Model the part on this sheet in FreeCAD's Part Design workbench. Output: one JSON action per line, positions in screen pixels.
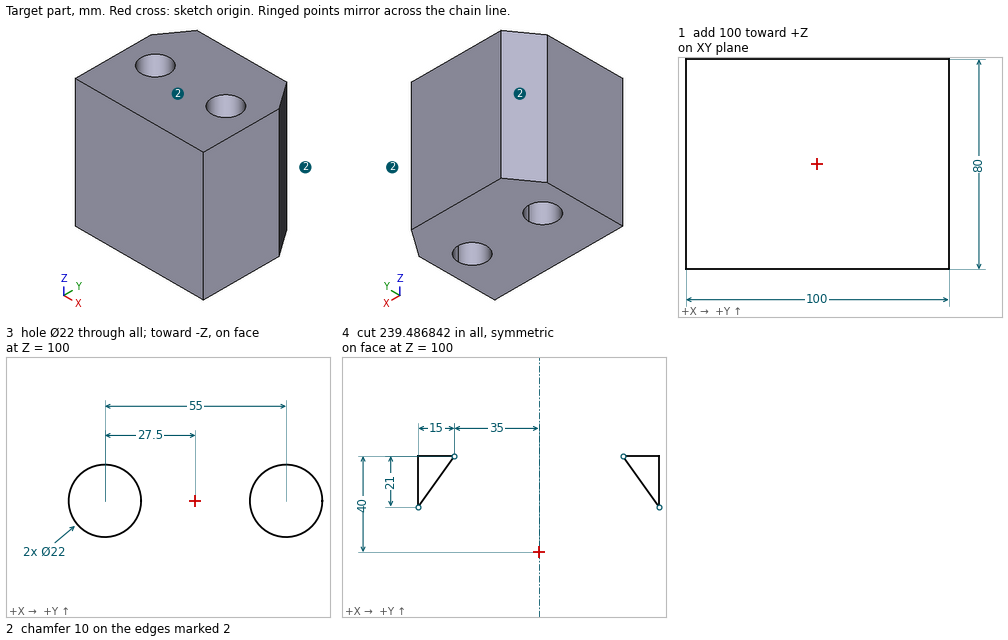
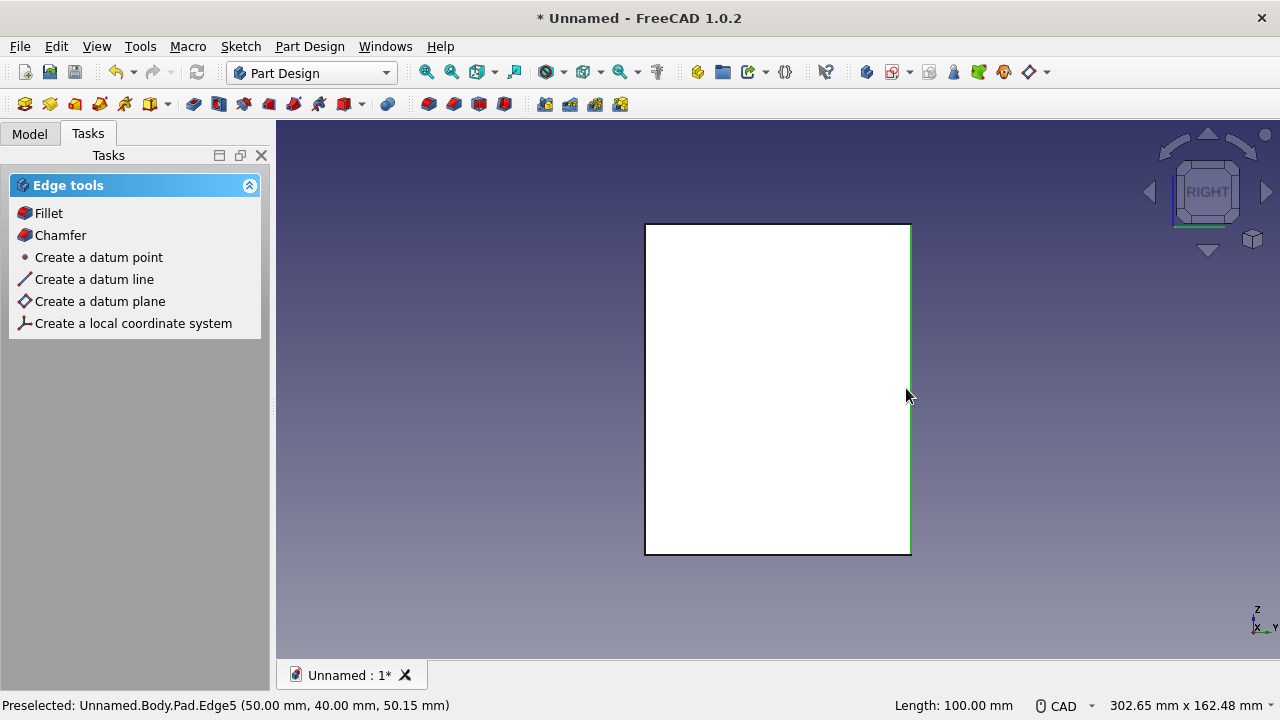
{"action": "key", "text": "5"}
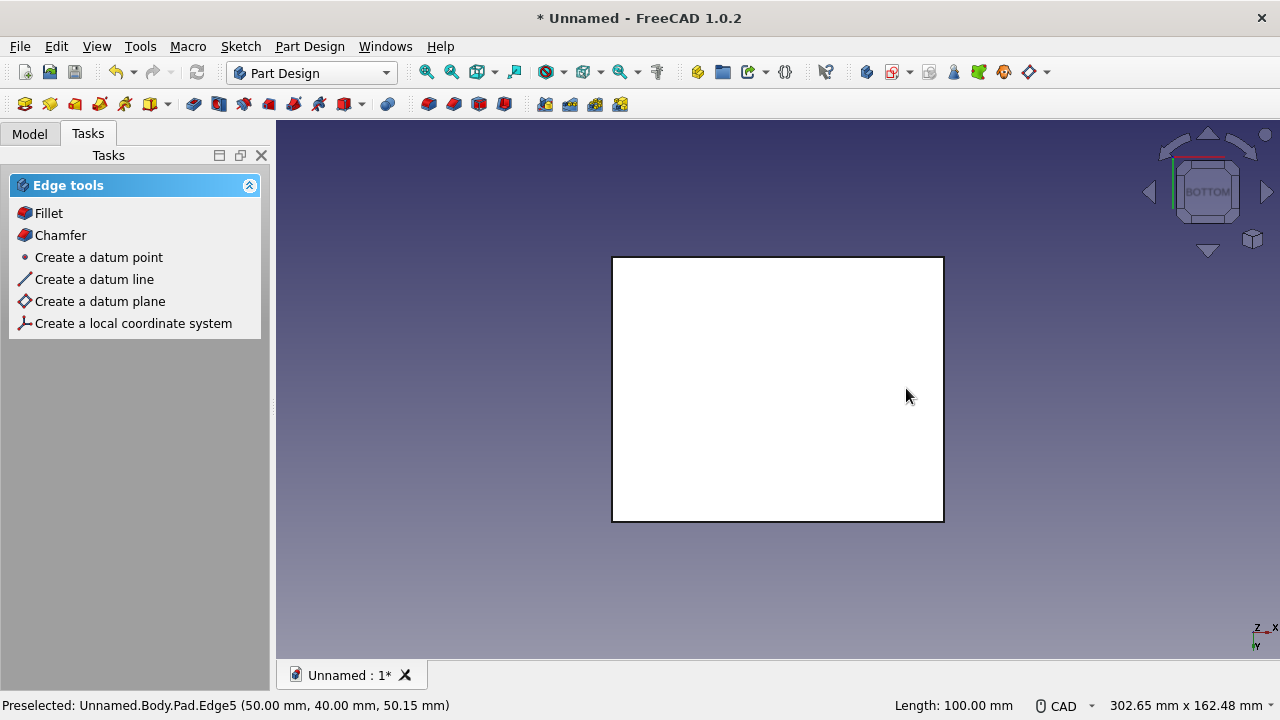
{"action": "key", "text": "4"}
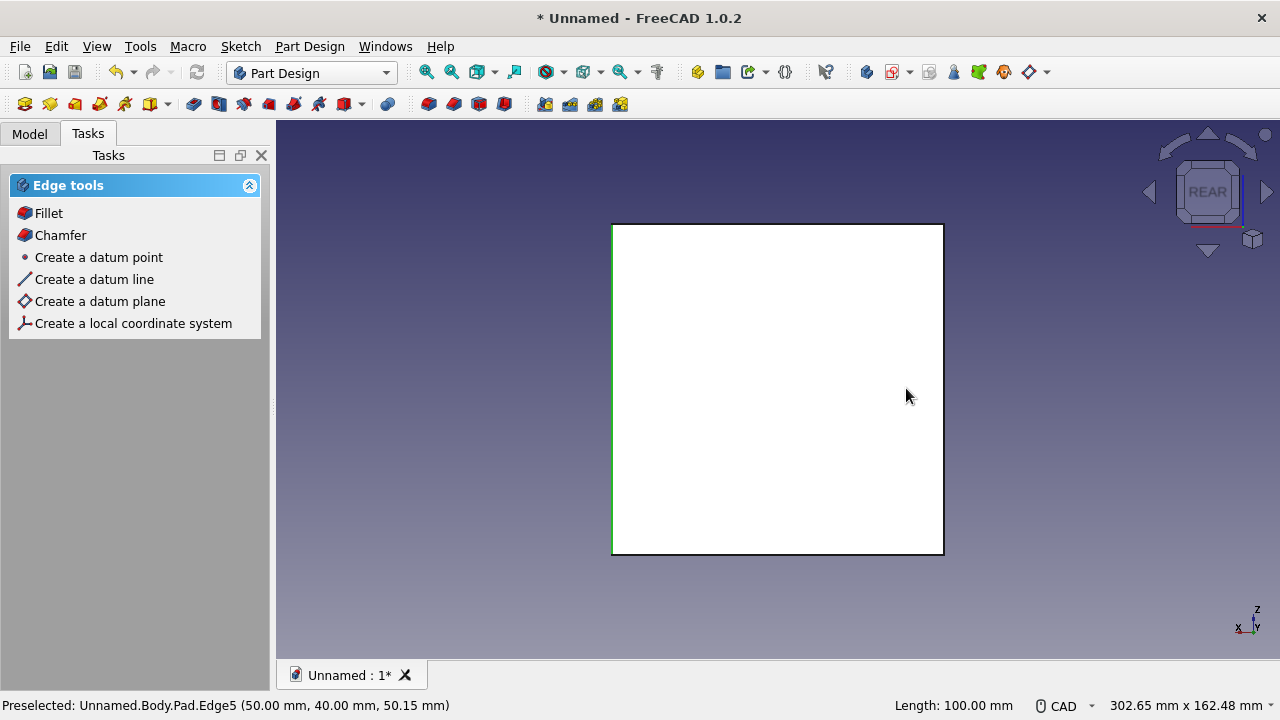
{"action": "left_click", "coordinate": [944, 388], "text": "ctrl"}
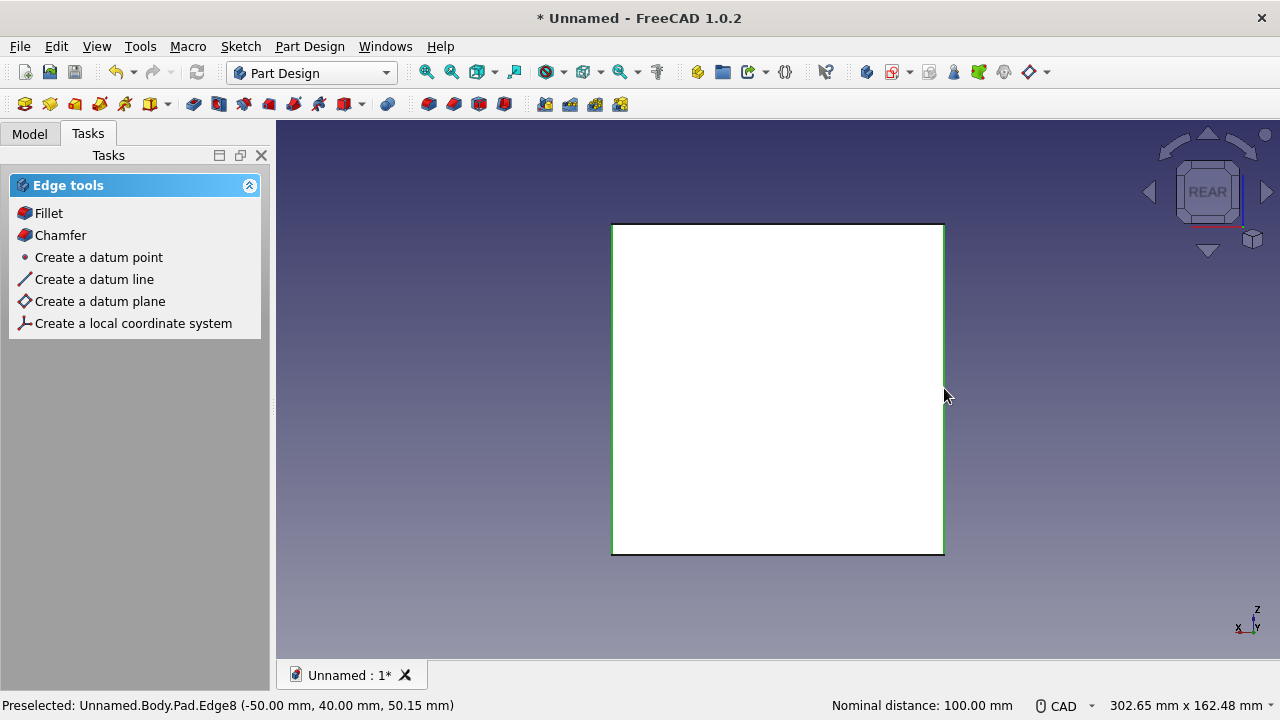
{"action": "left_click", "coordinate": [454, 104]}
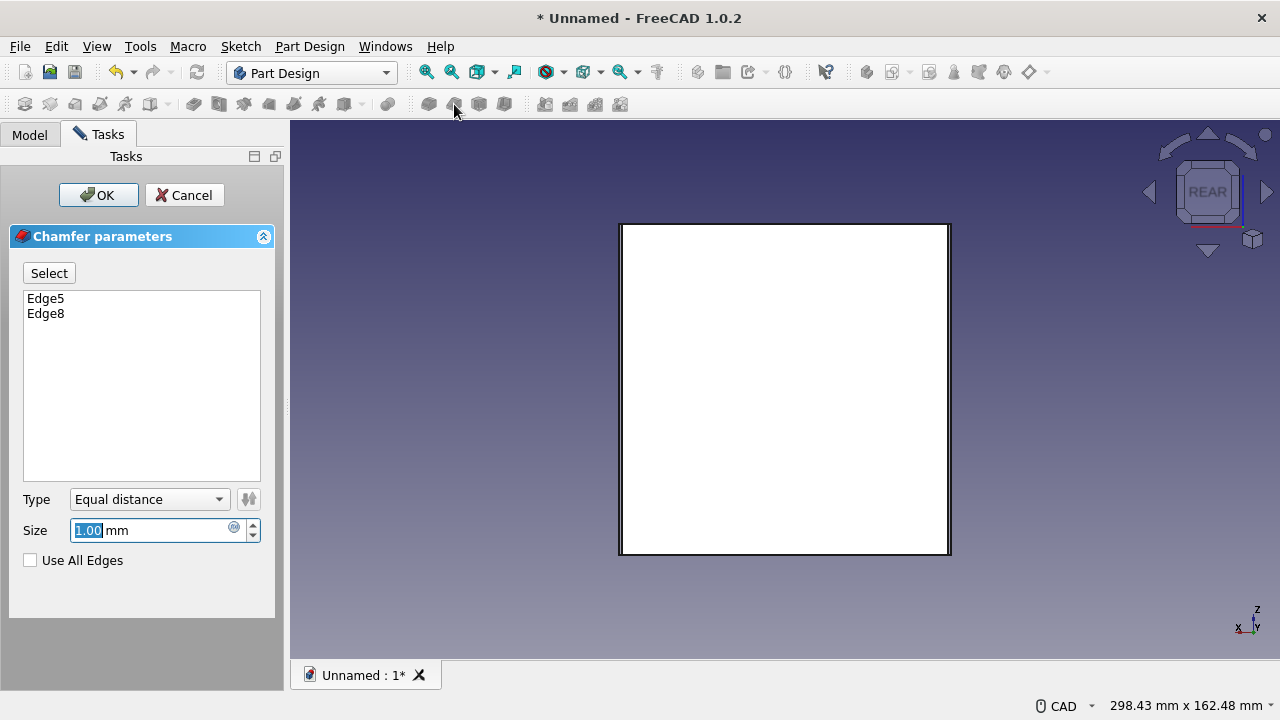
{"action": "type", "text": "10"}
{"action": "key", "text": "Tab"}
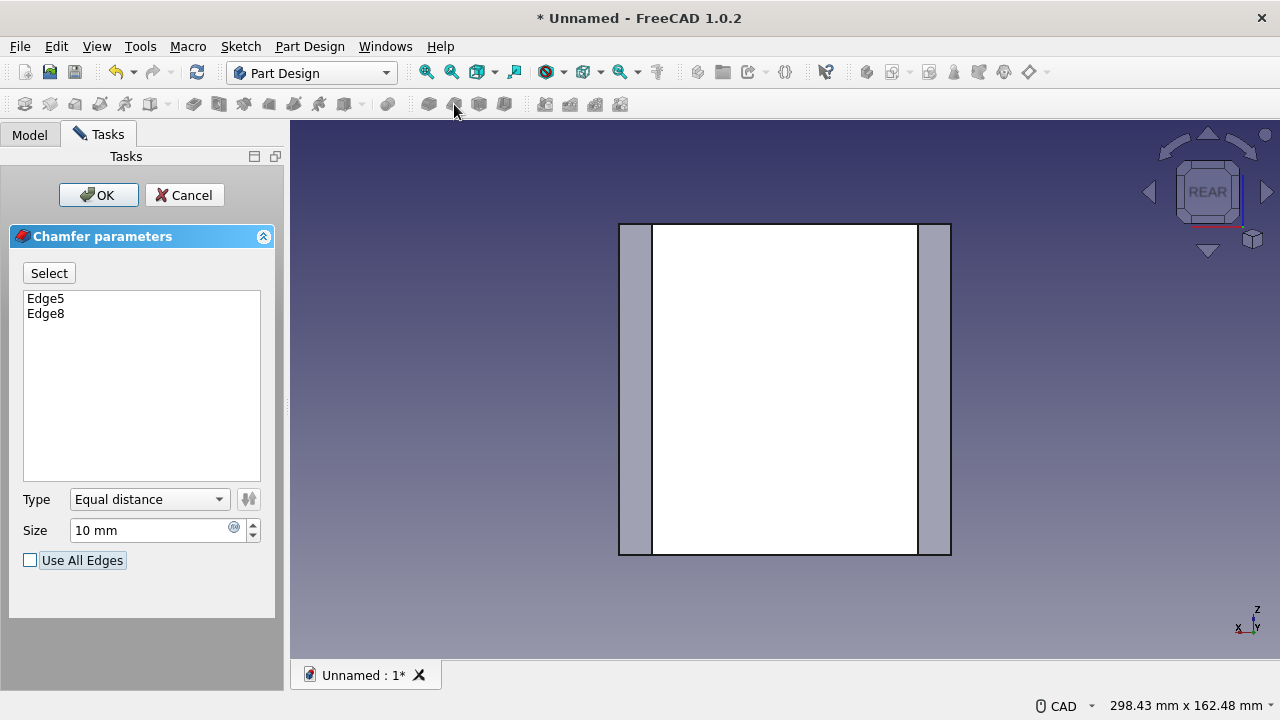
{"action": "left_click", "coordinate": [99, 195]}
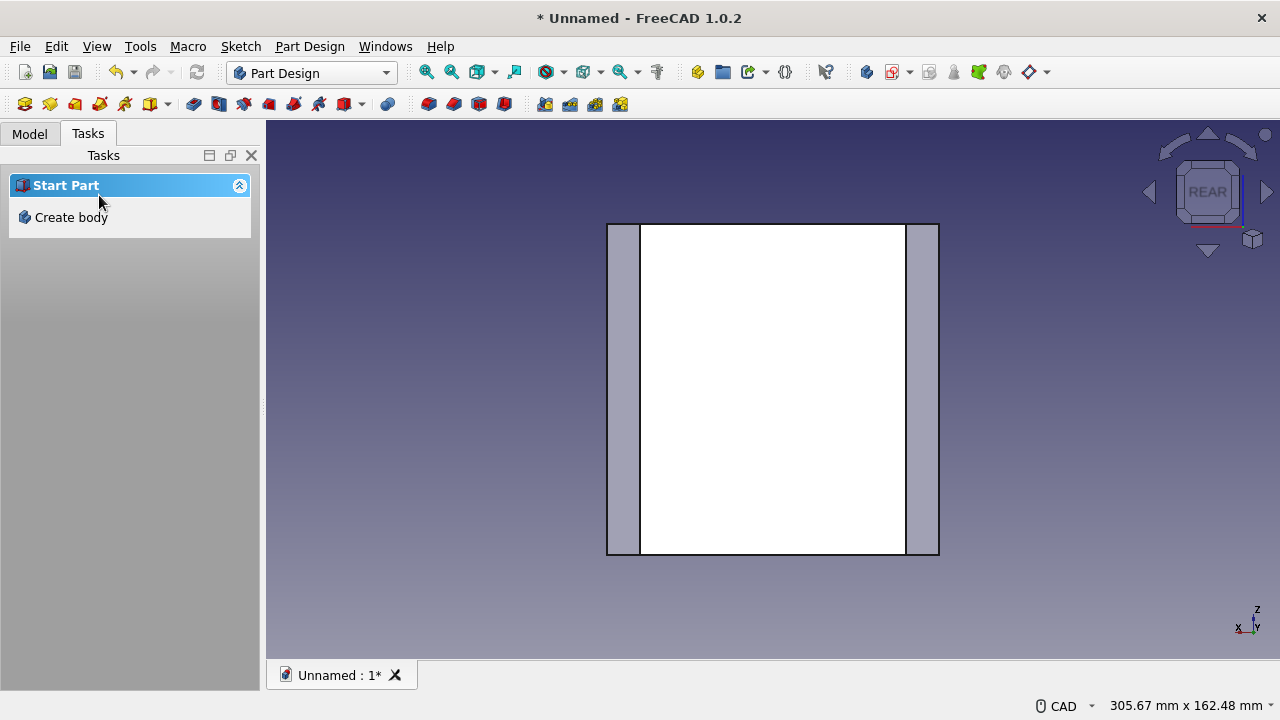
{"action": "key", "text": "0"}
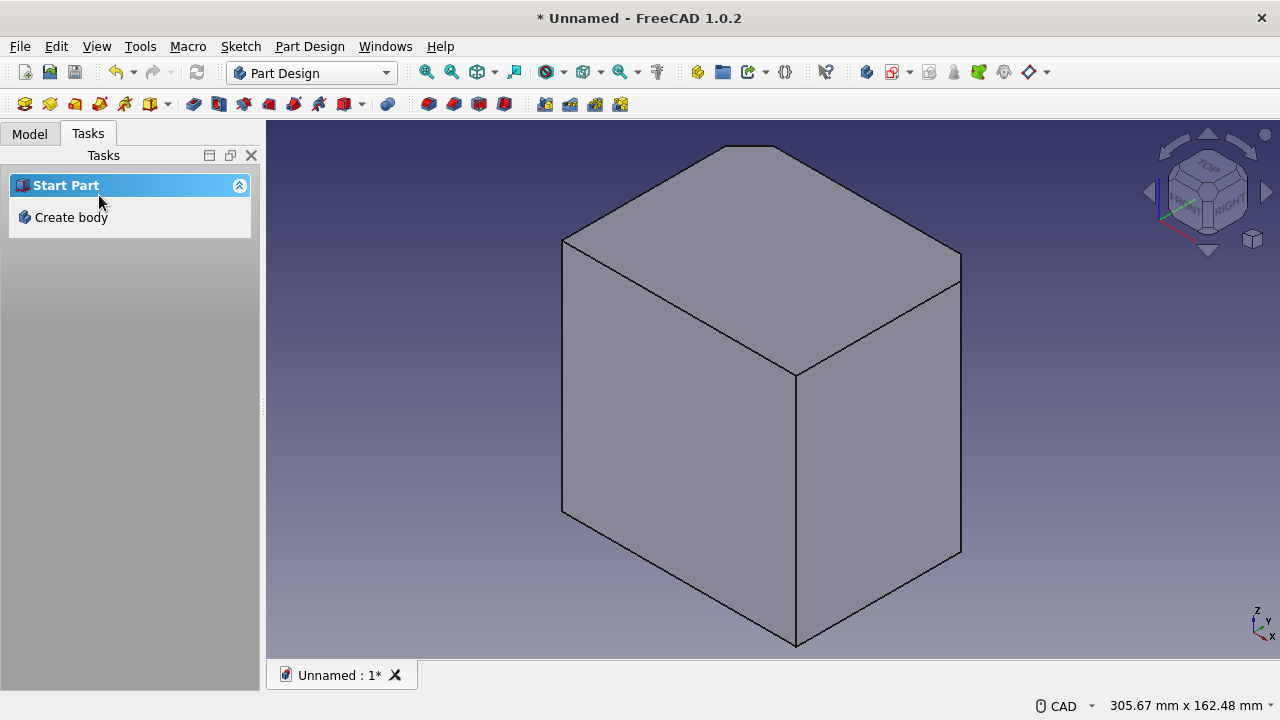
{"action": "left_click", "coordinate": [773, 253]}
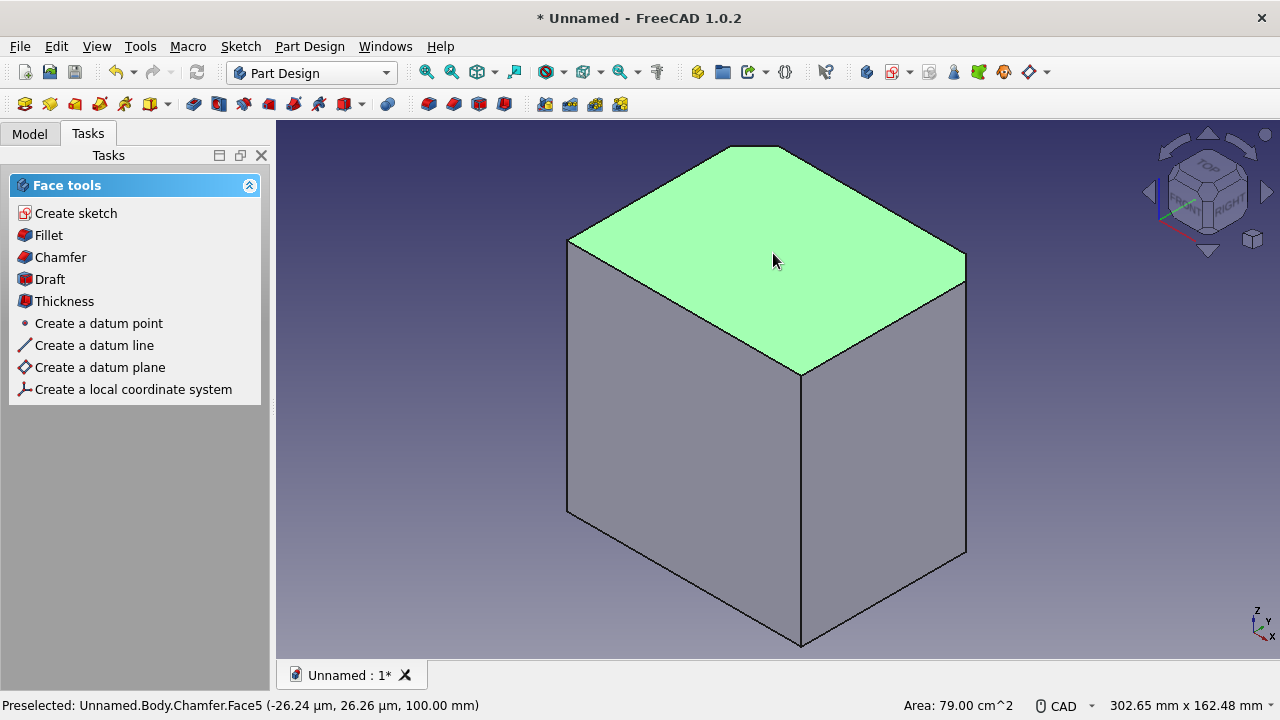
{"action": "left_click", "coordinate": [892, 72]}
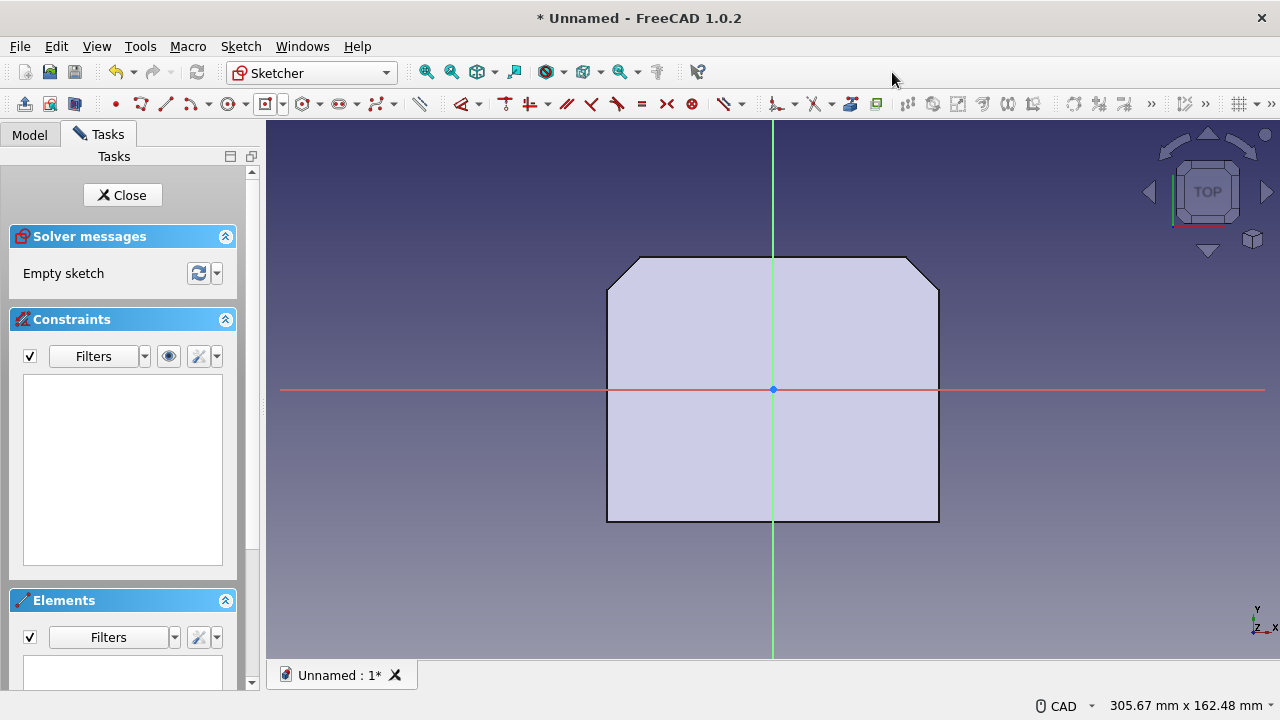
{"action": "scroll", "coordinate": [829, 390], "scroll_direction": "up", "scroll_amount": 4}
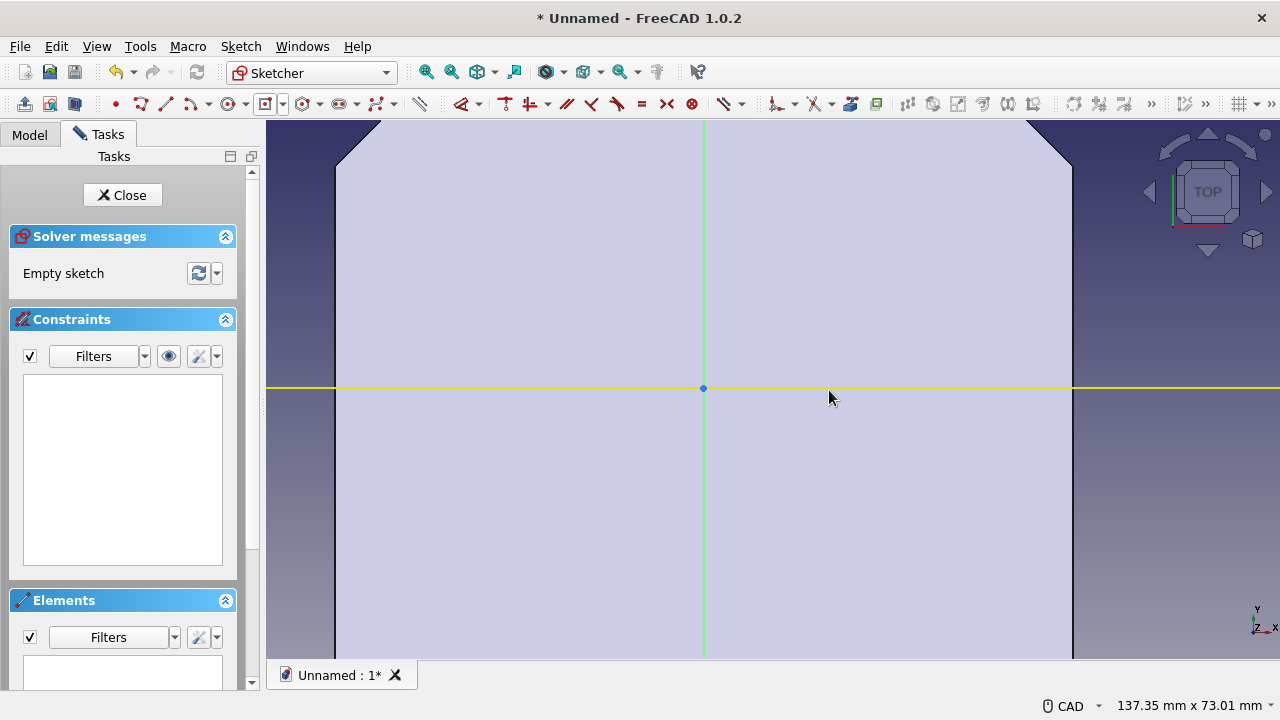
{"action": "left_click", "coordinate": [228, 104]}